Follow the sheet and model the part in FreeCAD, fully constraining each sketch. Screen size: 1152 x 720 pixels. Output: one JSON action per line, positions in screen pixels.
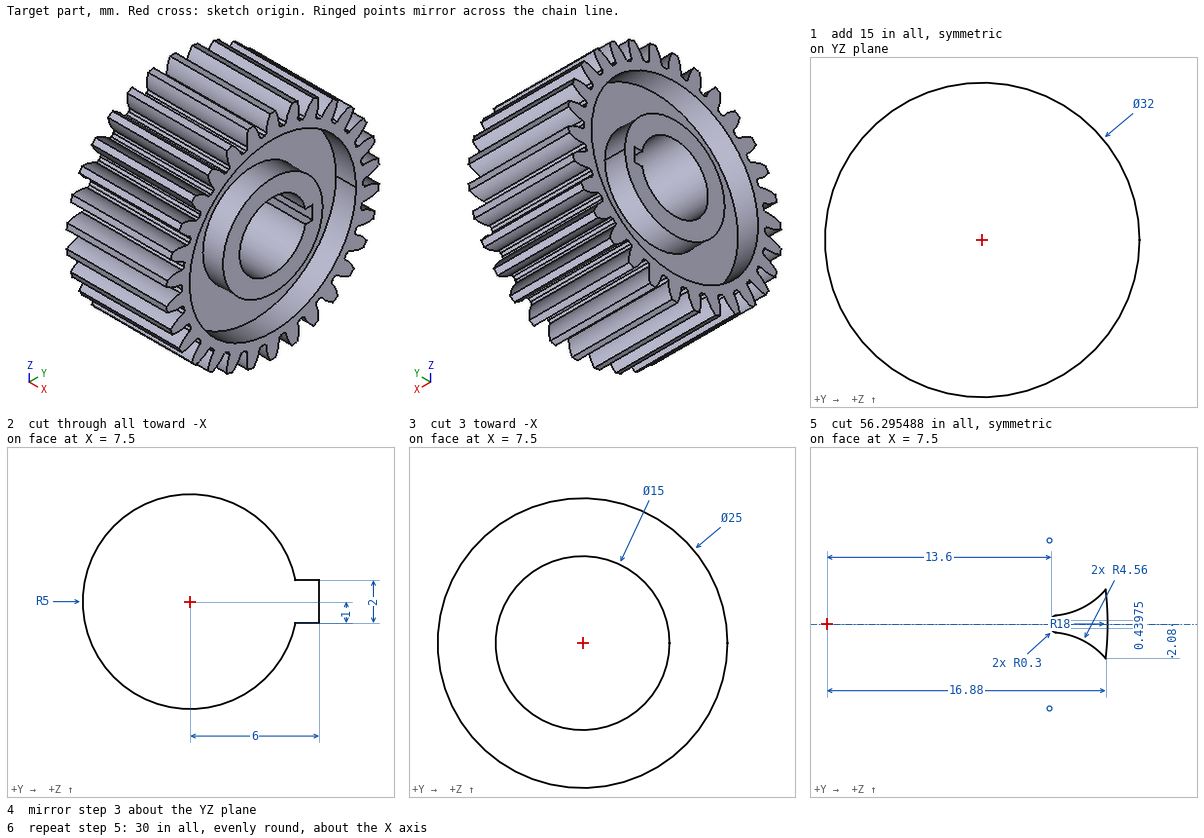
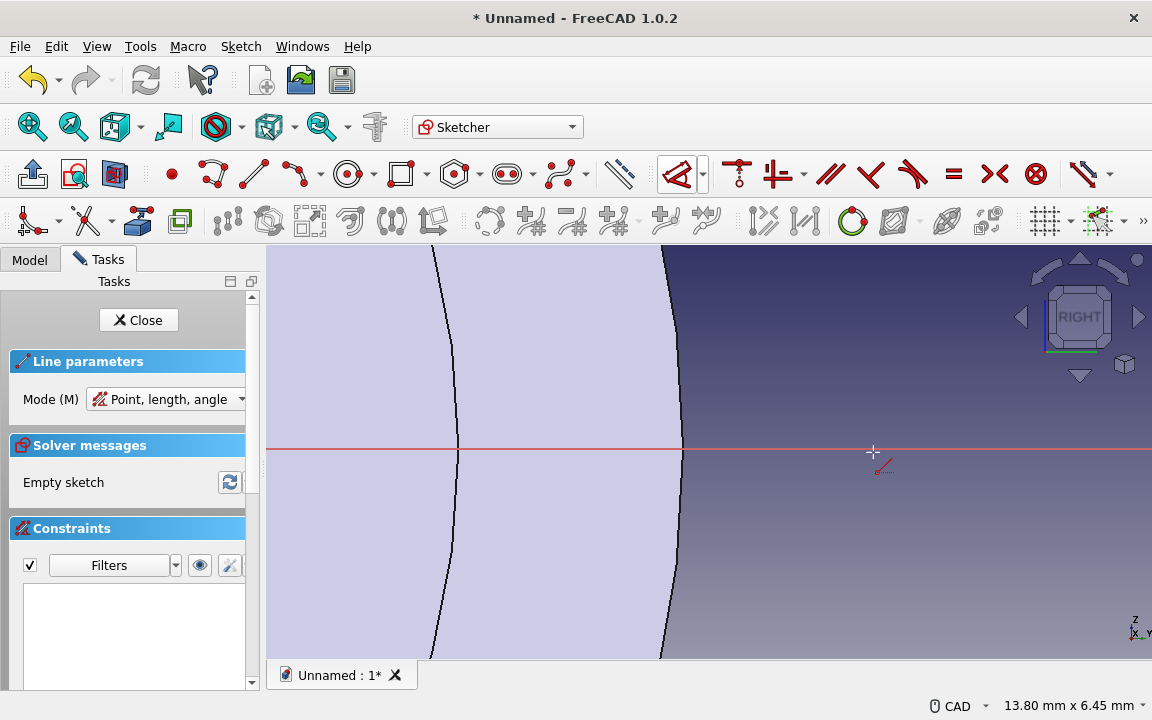
{"action": "left_click", "coordinate": [529, 435]}
{"action": "left_click", "coordinate": [529, 463]}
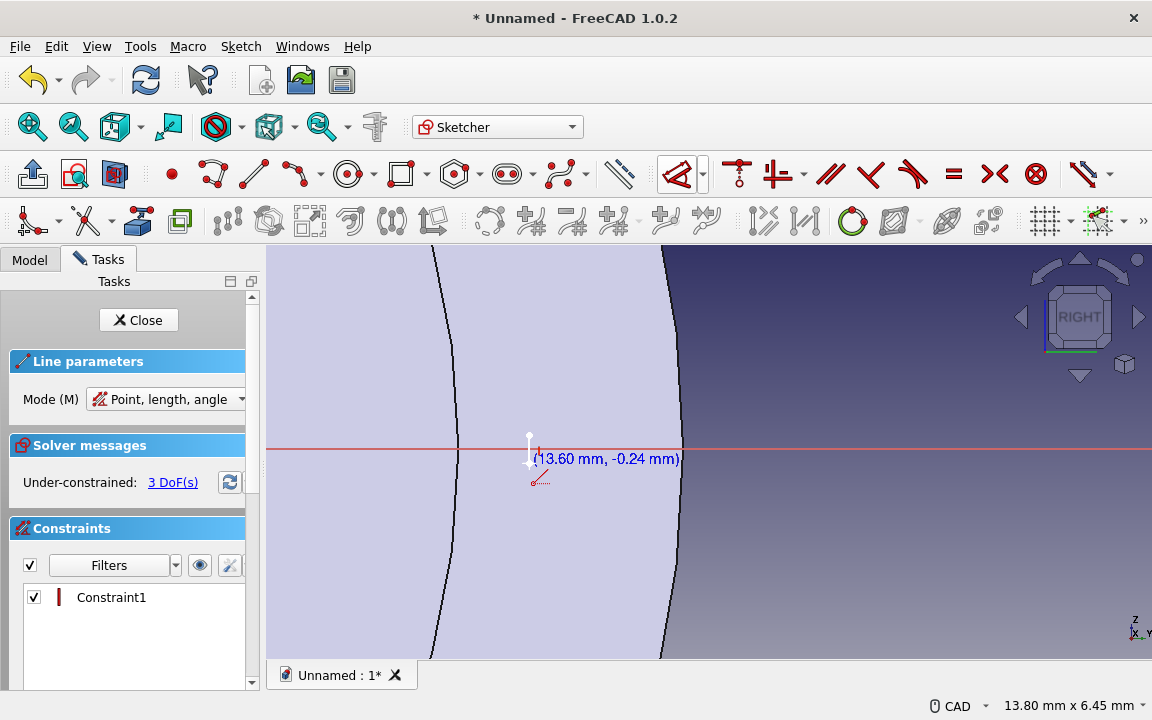
{"action": "key", "text": "g 3 a"}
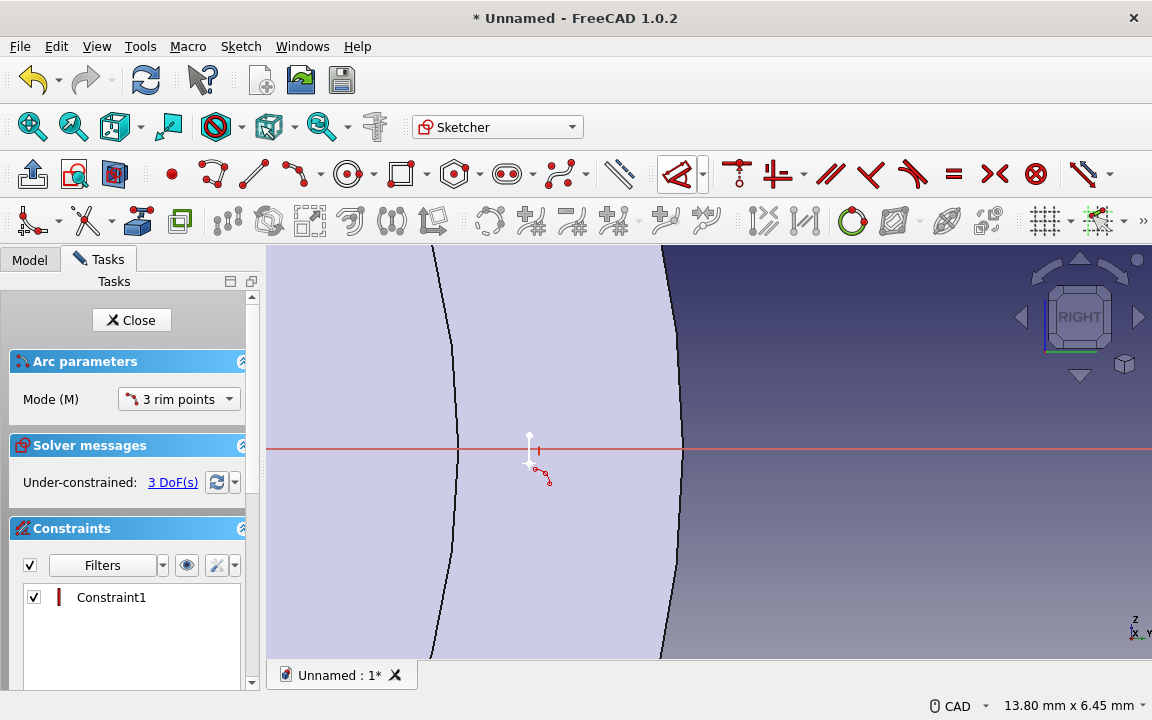
{"action": "left_click", "coordinate": [529, 464]}
{"action": "left_click", "coordinate": [546, 482]}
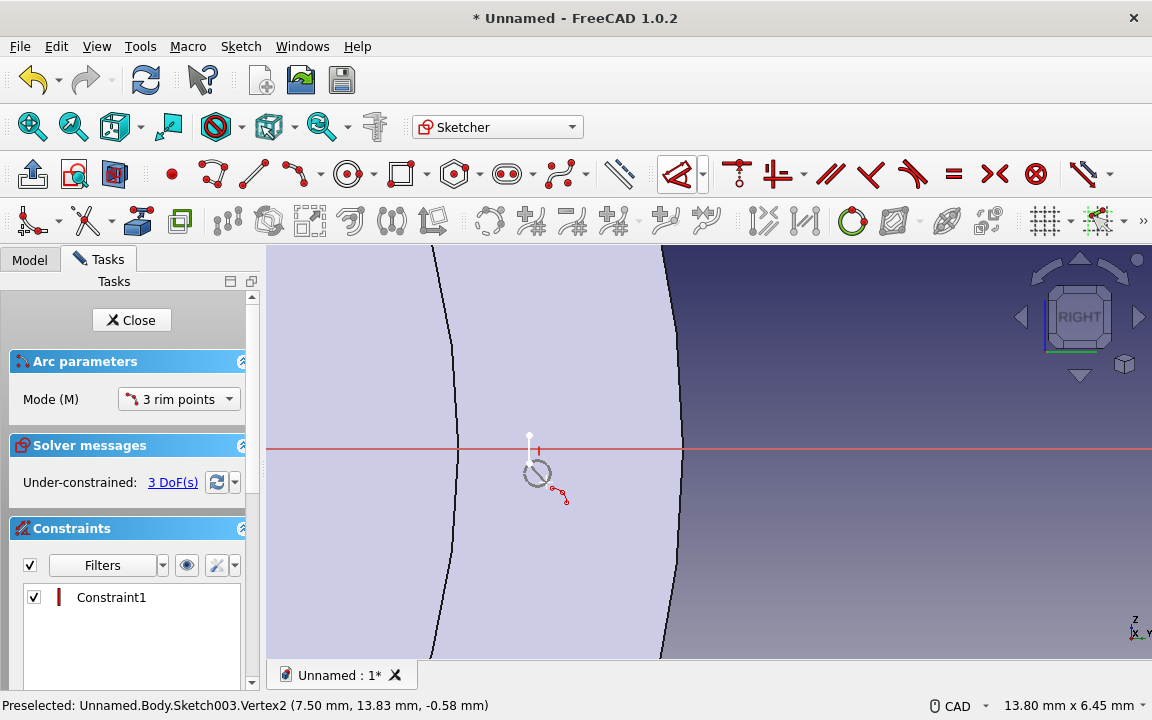
{"action": "scroll", "coordinate": [534, 476], "scroll_direction": "up", "scroll_amount": 6}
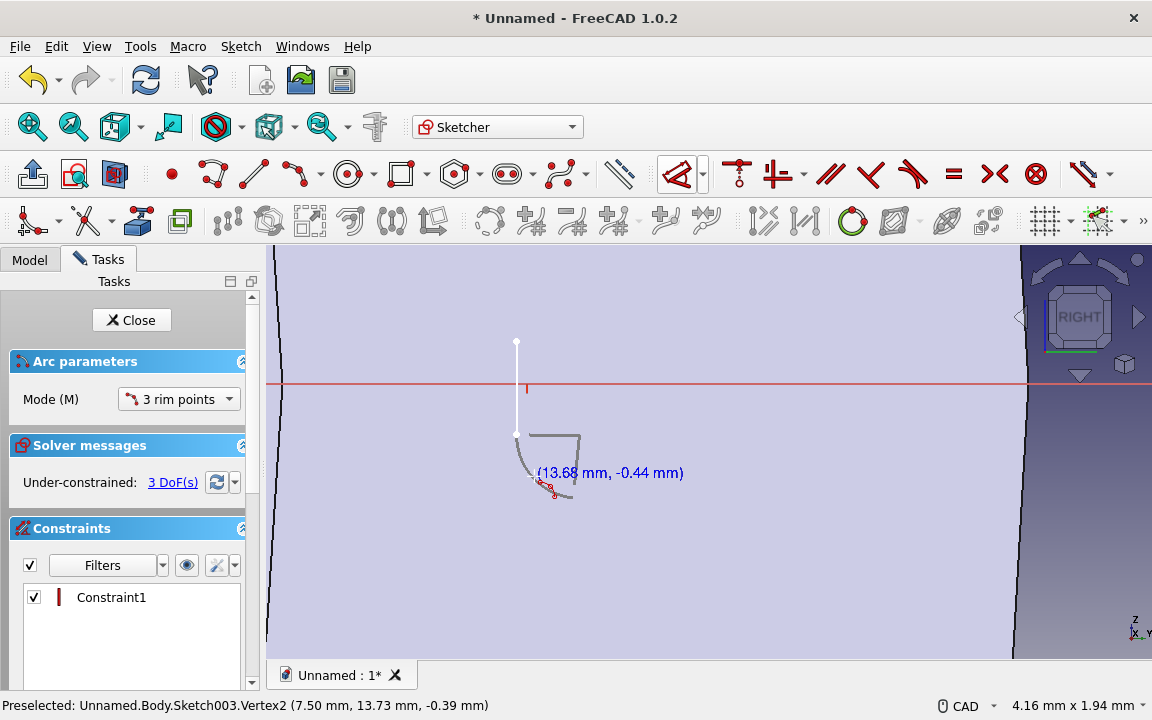
{"action": "left_click", "coordinate": [534, 474]}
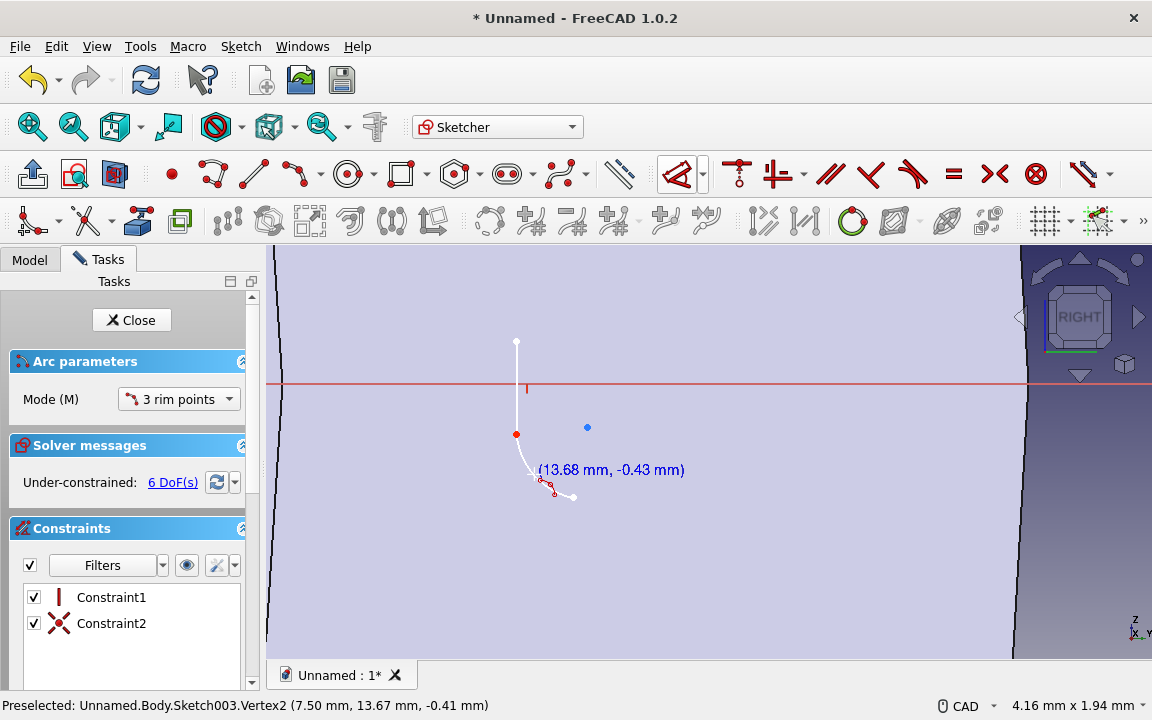
{"action": "left_click", "coordinate": [573, 498]}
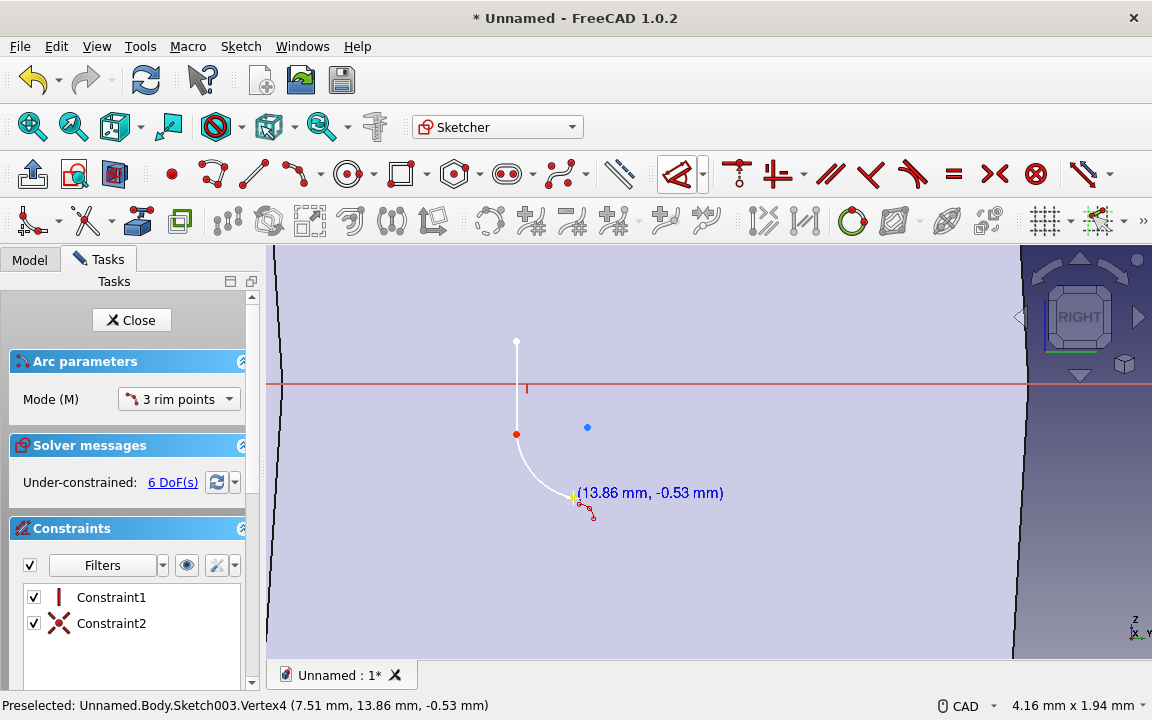
{"action": "scroll", "coordinate": [538, 481], "scroll_direction": "down", "scroll_amount": 6}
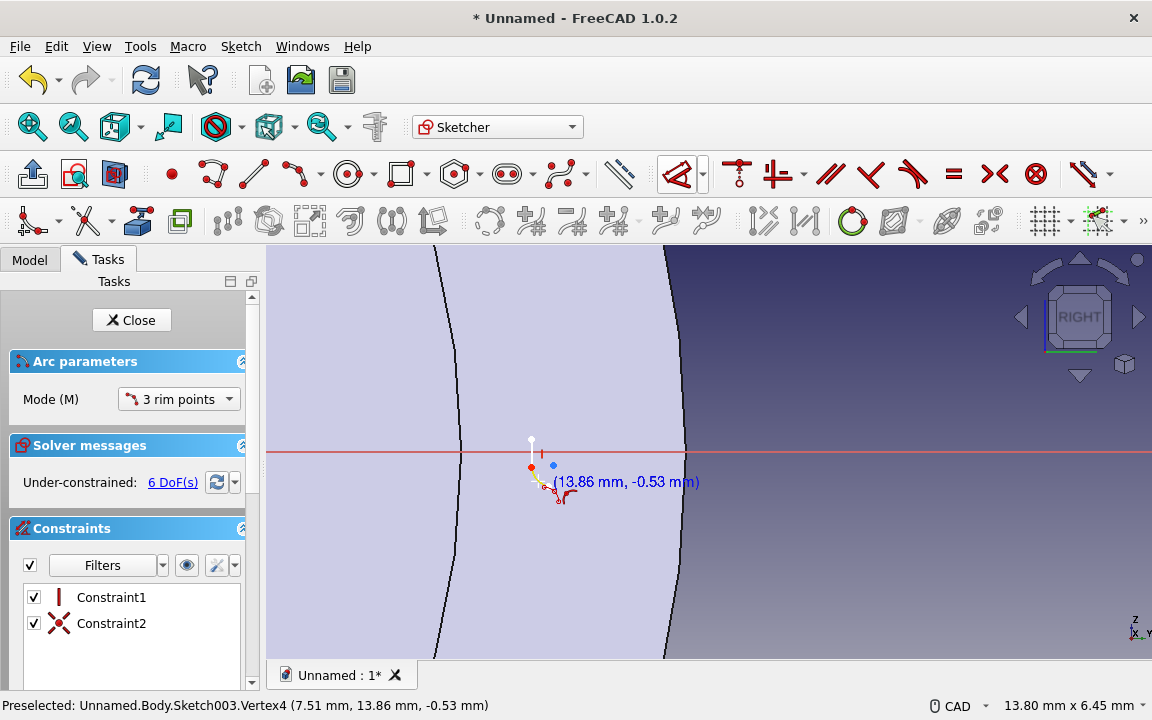
{"action": "left_click", "coordinate": [742, 586]}
{"action": "left_click", "coordinate": [656, 517]}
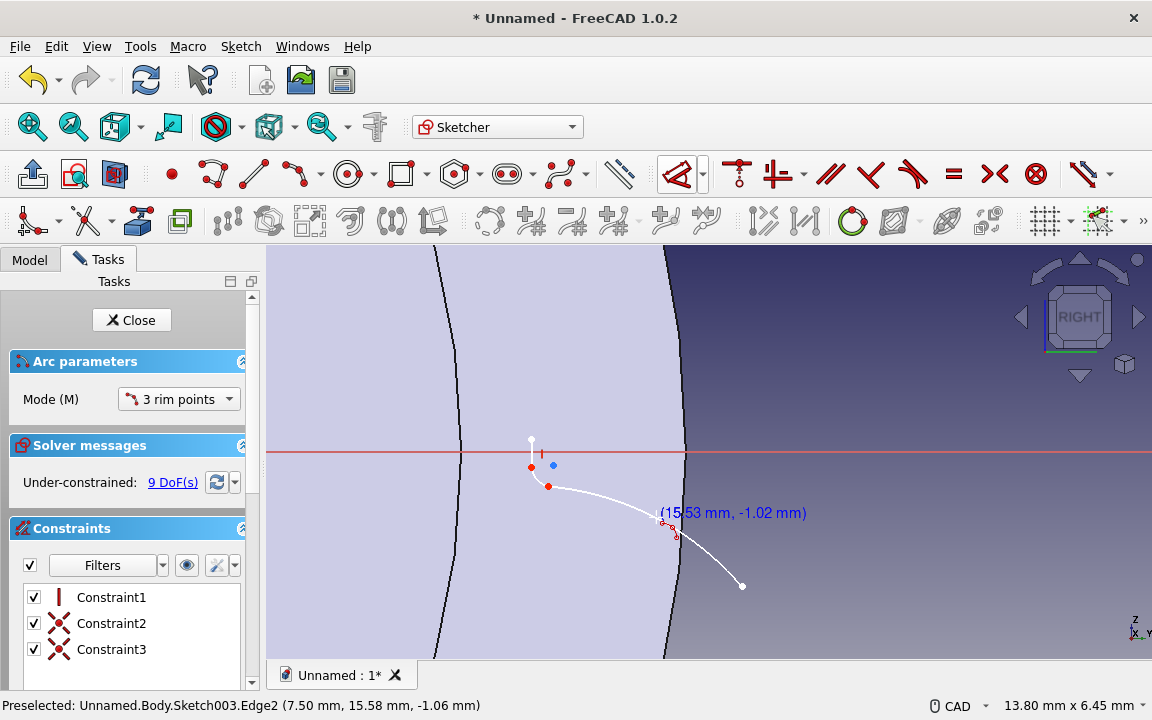
{"action": "left_click", "coordinate": [742, 587]}
{"action": "left_click", "coordinate": [742, 319]}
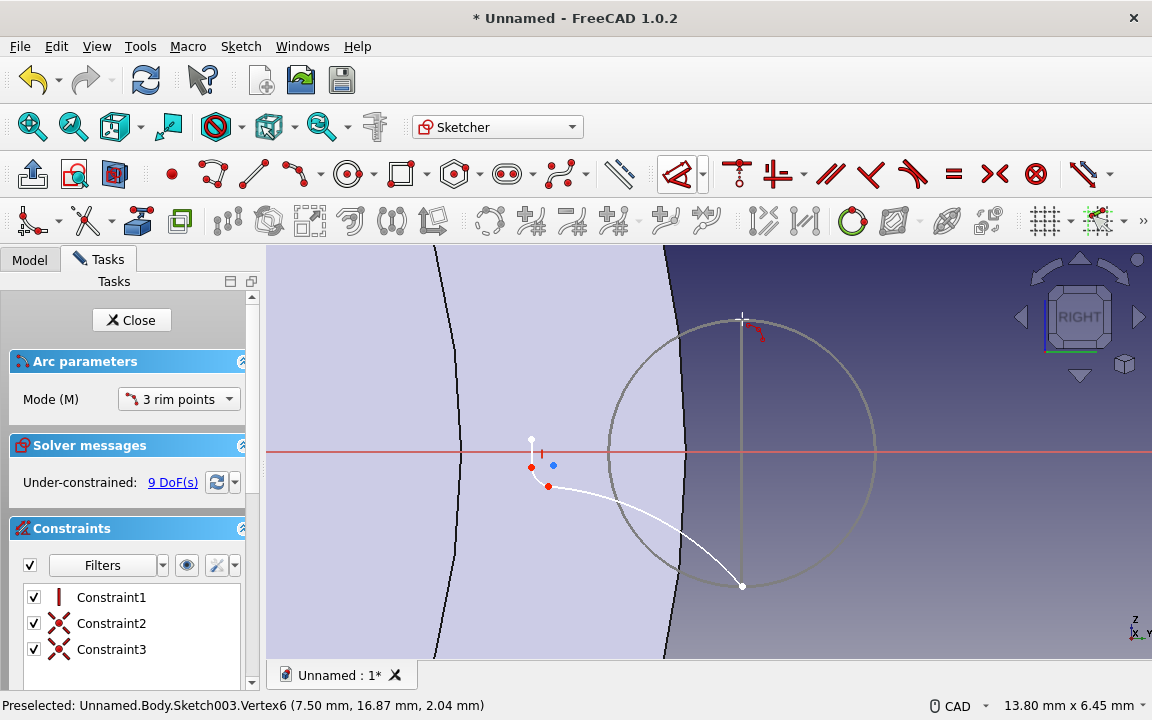
{"action": "scroll", "coordinate": [750, 479], "scroll_direction": "up", "scroll_amount": 4}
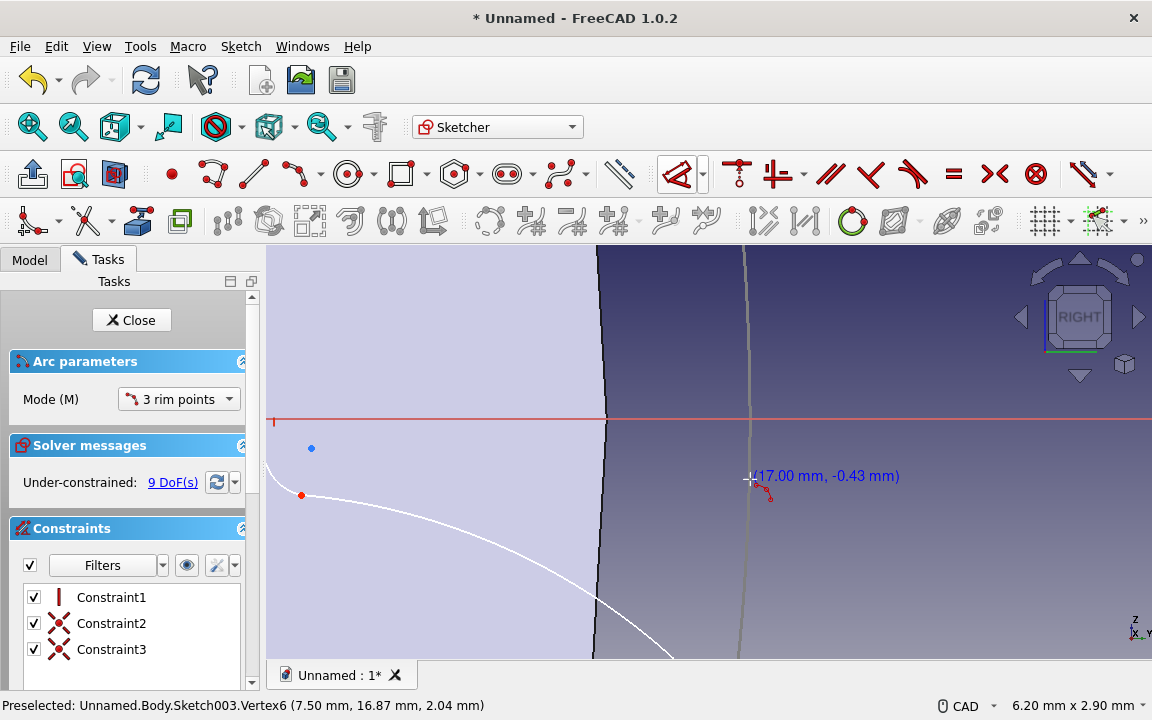
{"action": "left_click", "coordinate": [749, 478]}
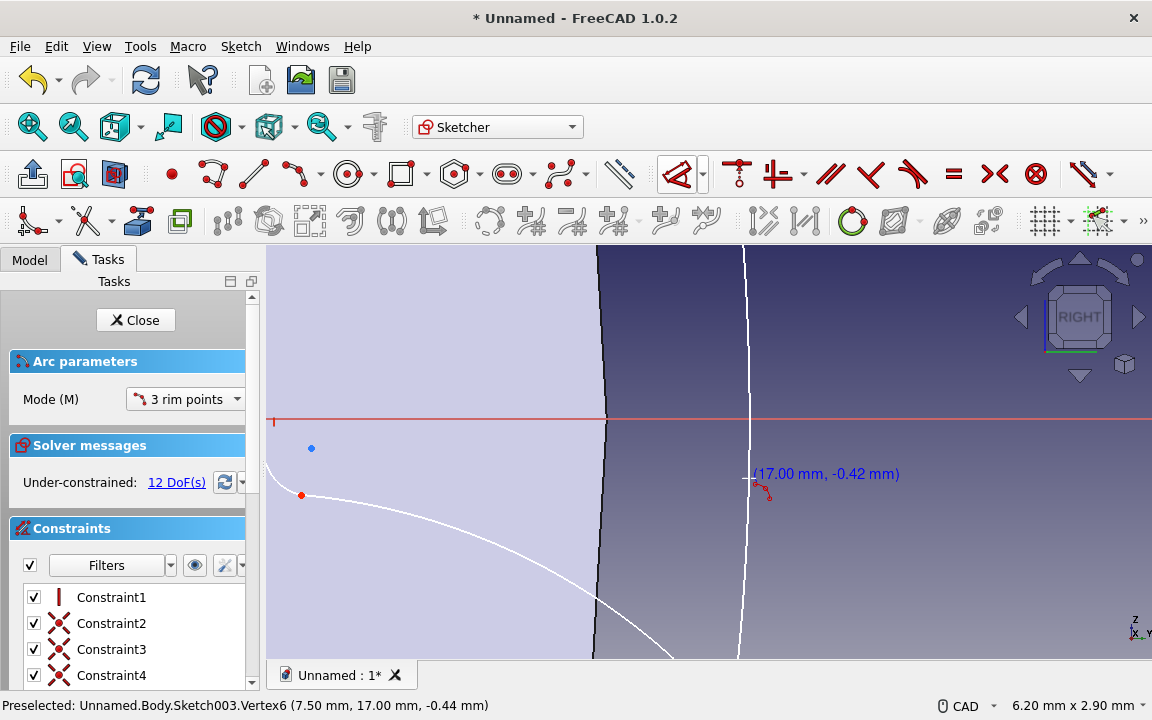
{"action": "scroll", "coordinate": [750, 479], "scroll_direction": "down", "scroll_amount": 4}